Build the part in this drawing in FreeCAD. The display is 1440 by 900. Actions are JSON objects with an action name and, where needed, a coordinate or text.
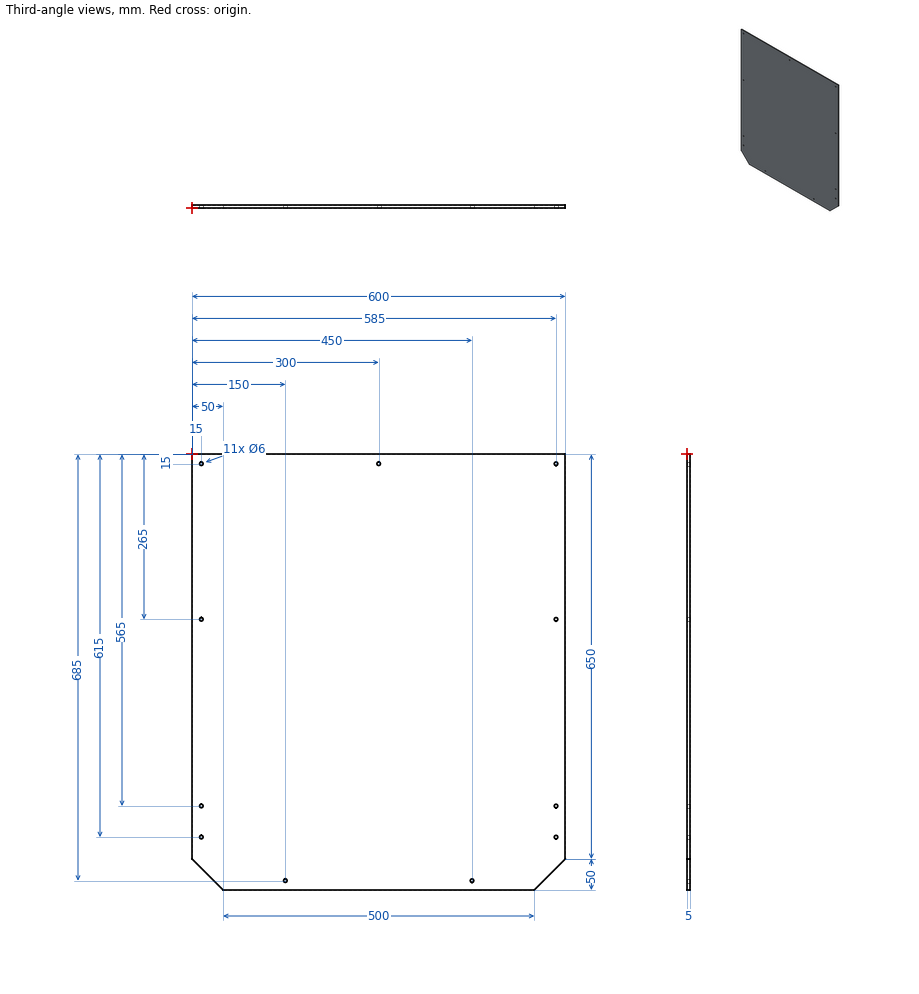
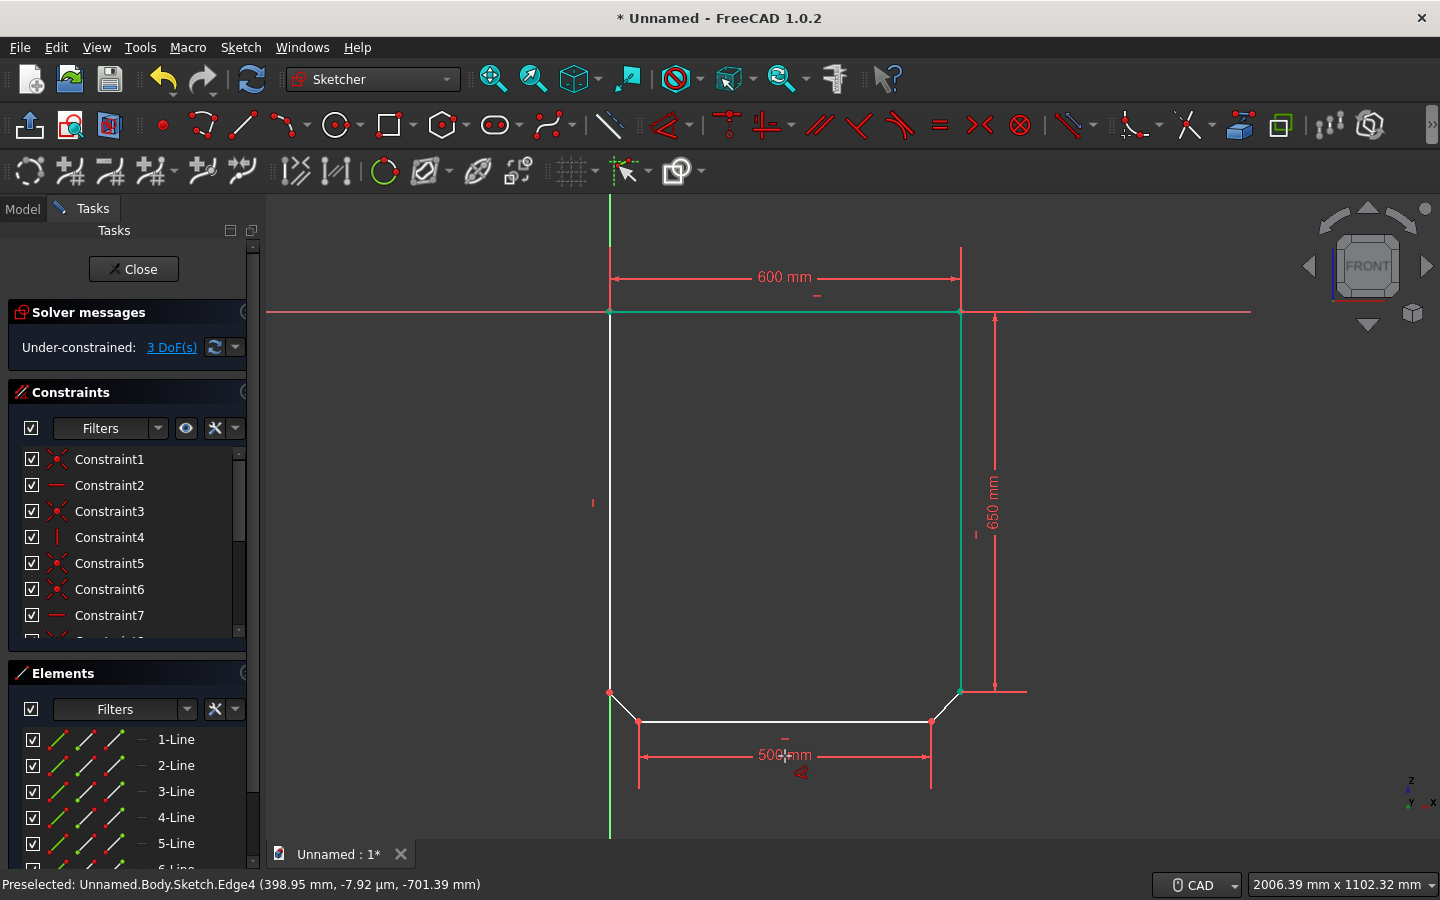
{"action": "left_click", "coordinate": [610, 579]}
{"action": "left_click", "coordinate": [576, 502]}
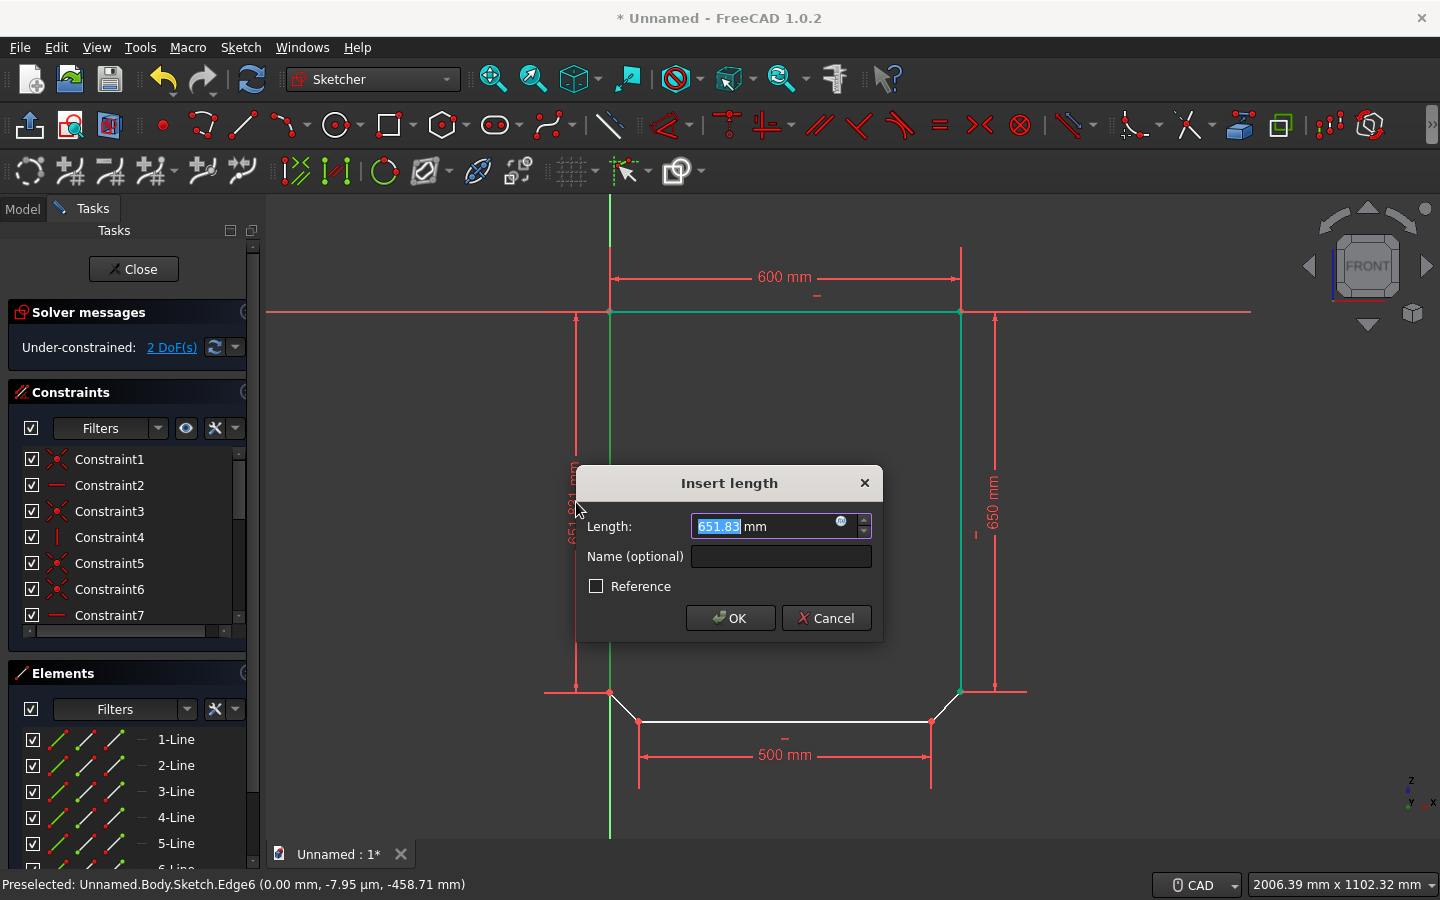
{"action": "type", "text": "650"}
{"action": "key", "text": "Return"}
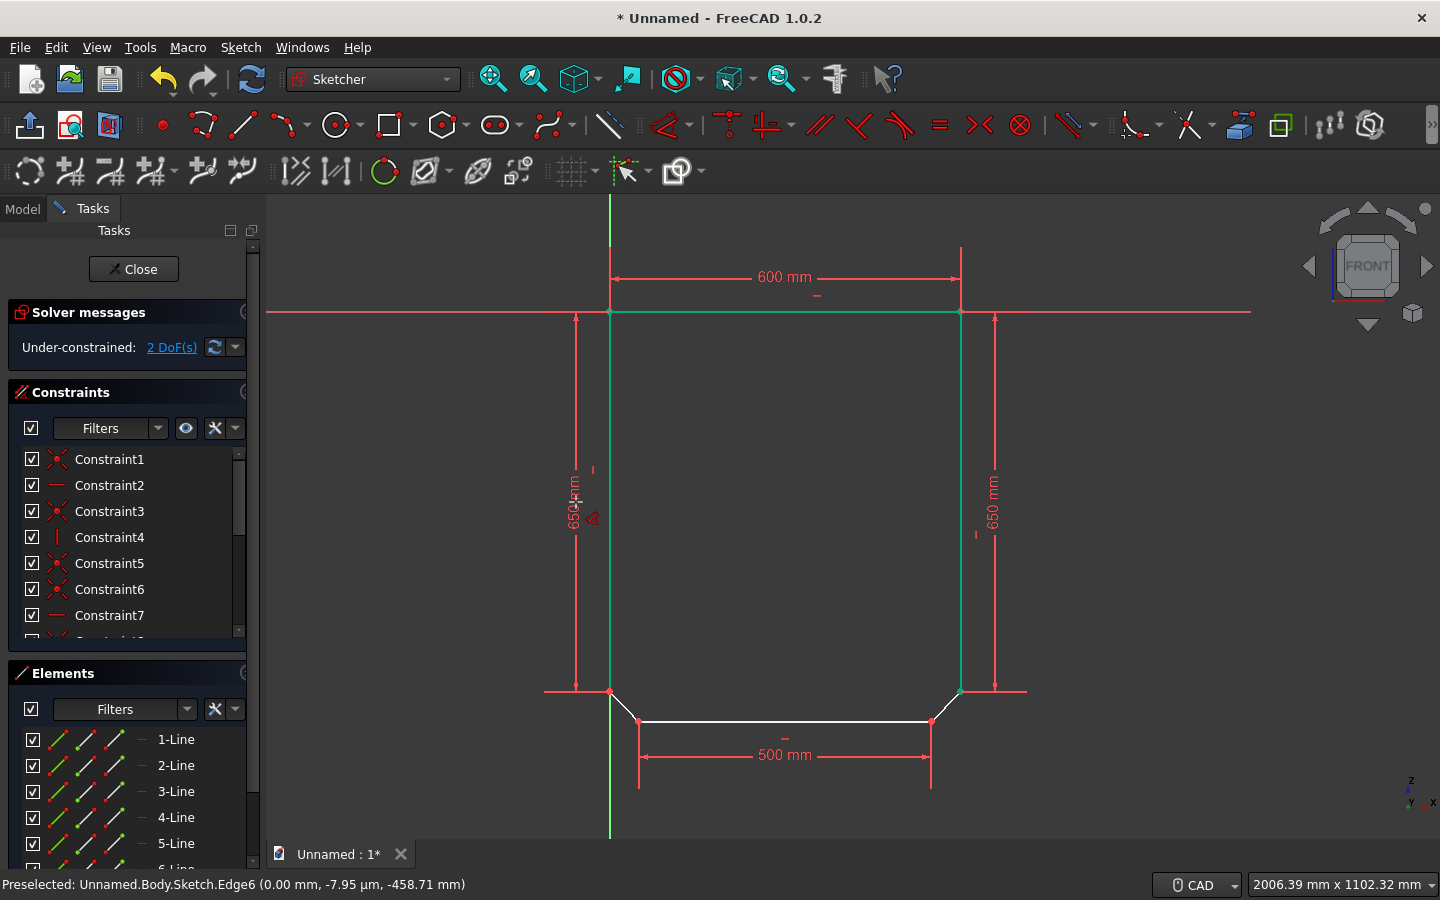
{"action": "scroll", "coordinate": [639, 722], "scroll_direction": "up", "scroll_amount": 2}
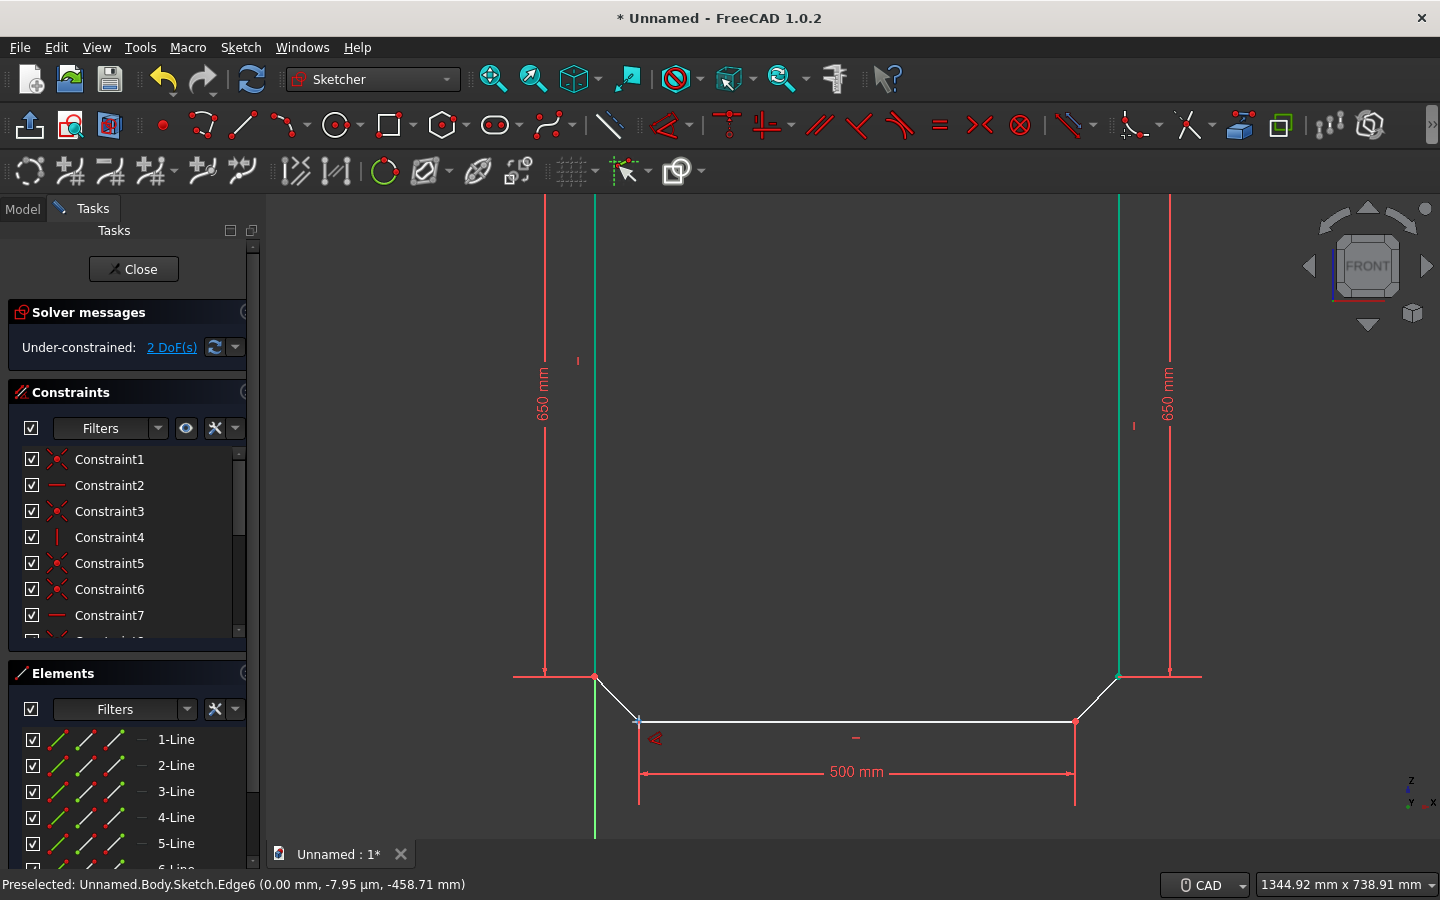
{"action": "left_click", "coordinate": [639, 722]}
{"action": "left_click", "coordinate": [617, 756]}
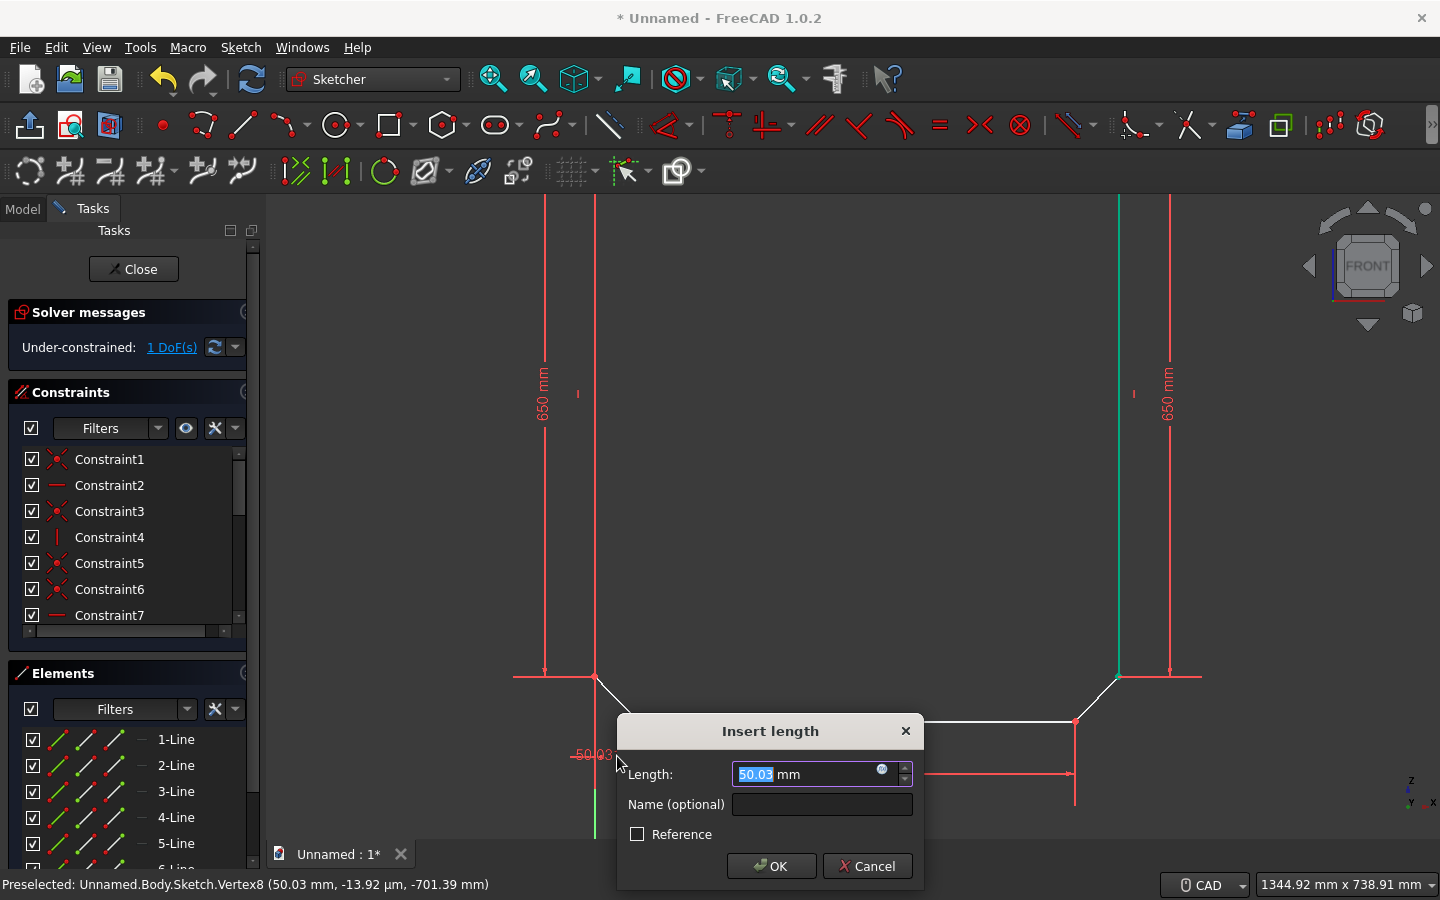
{"action": "type", "text": "50"}
{"action": "key", "text": "Return"}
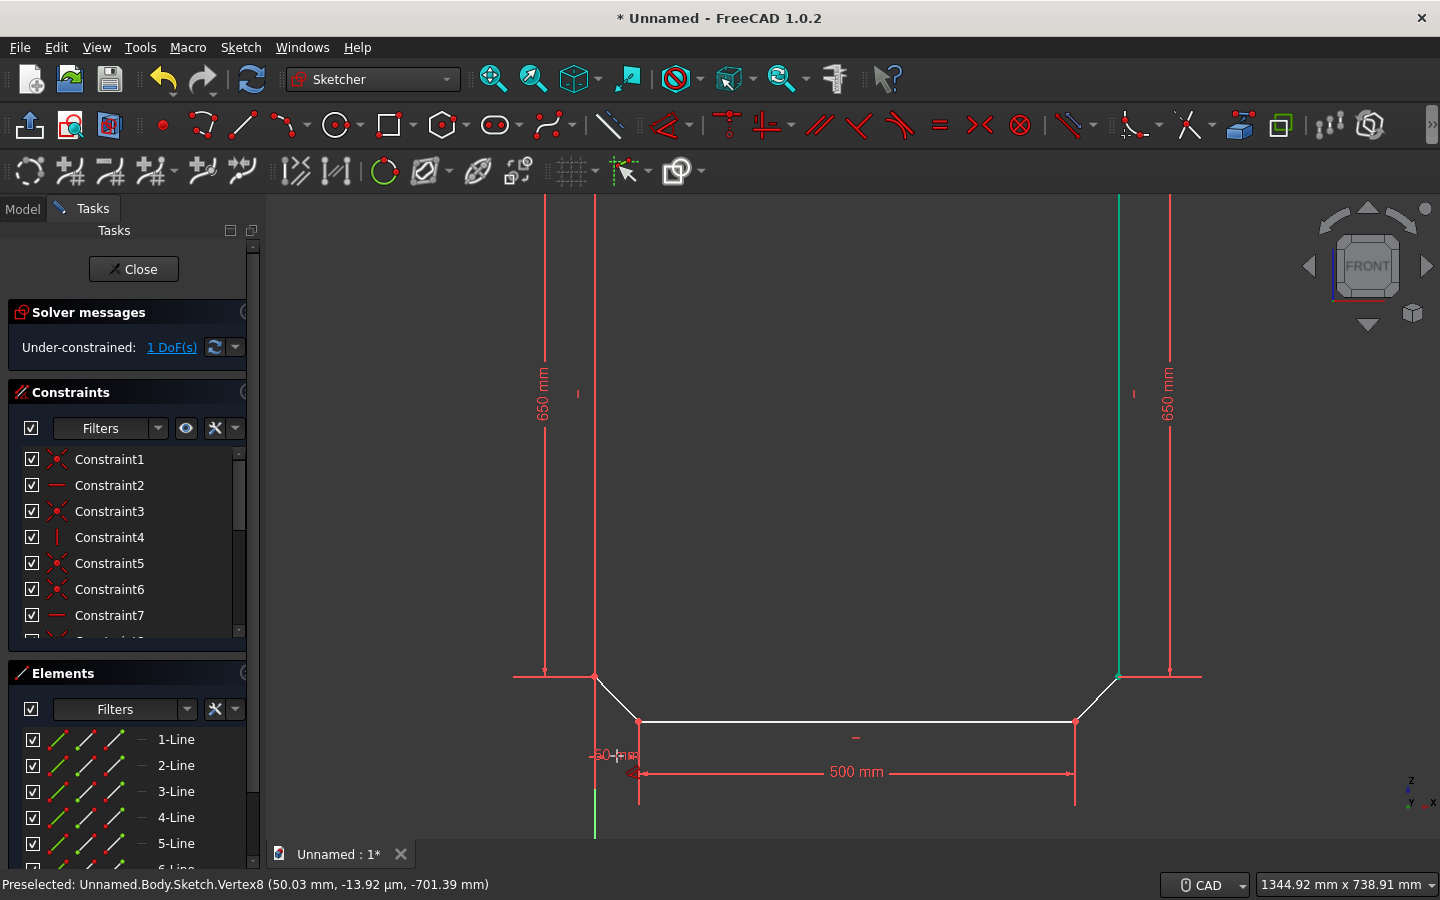
{"action": "left_click", "coordinate": [1106, 690]}
{"action": "left_click", "coordinate": [1153, 699]}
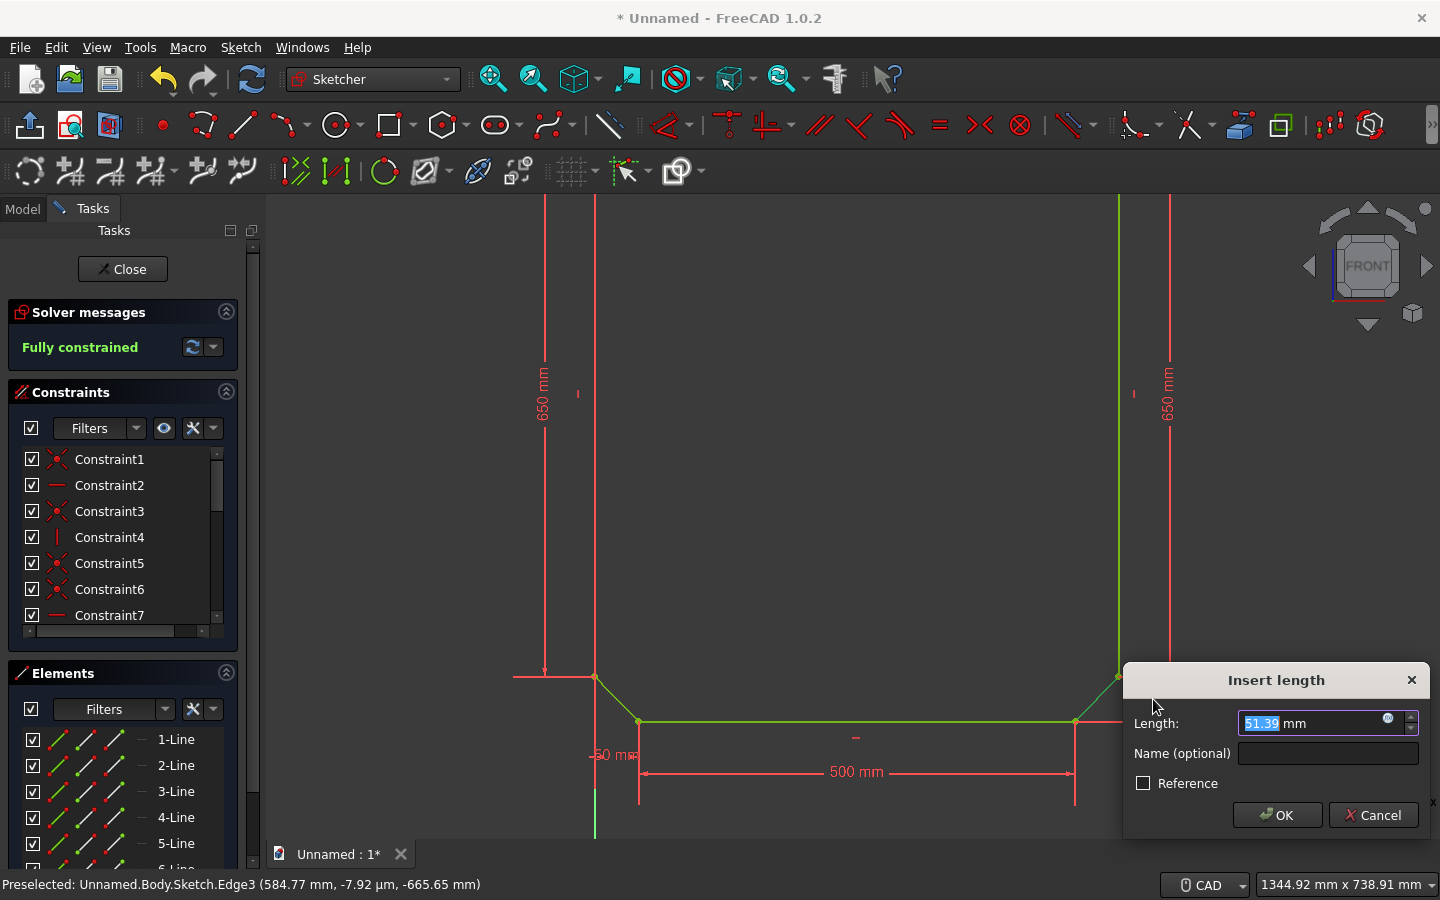
{"action": "type", "text": "50"}
{"action": "key", "text": "Return"}
{"action": "key", "text": "Escape"}